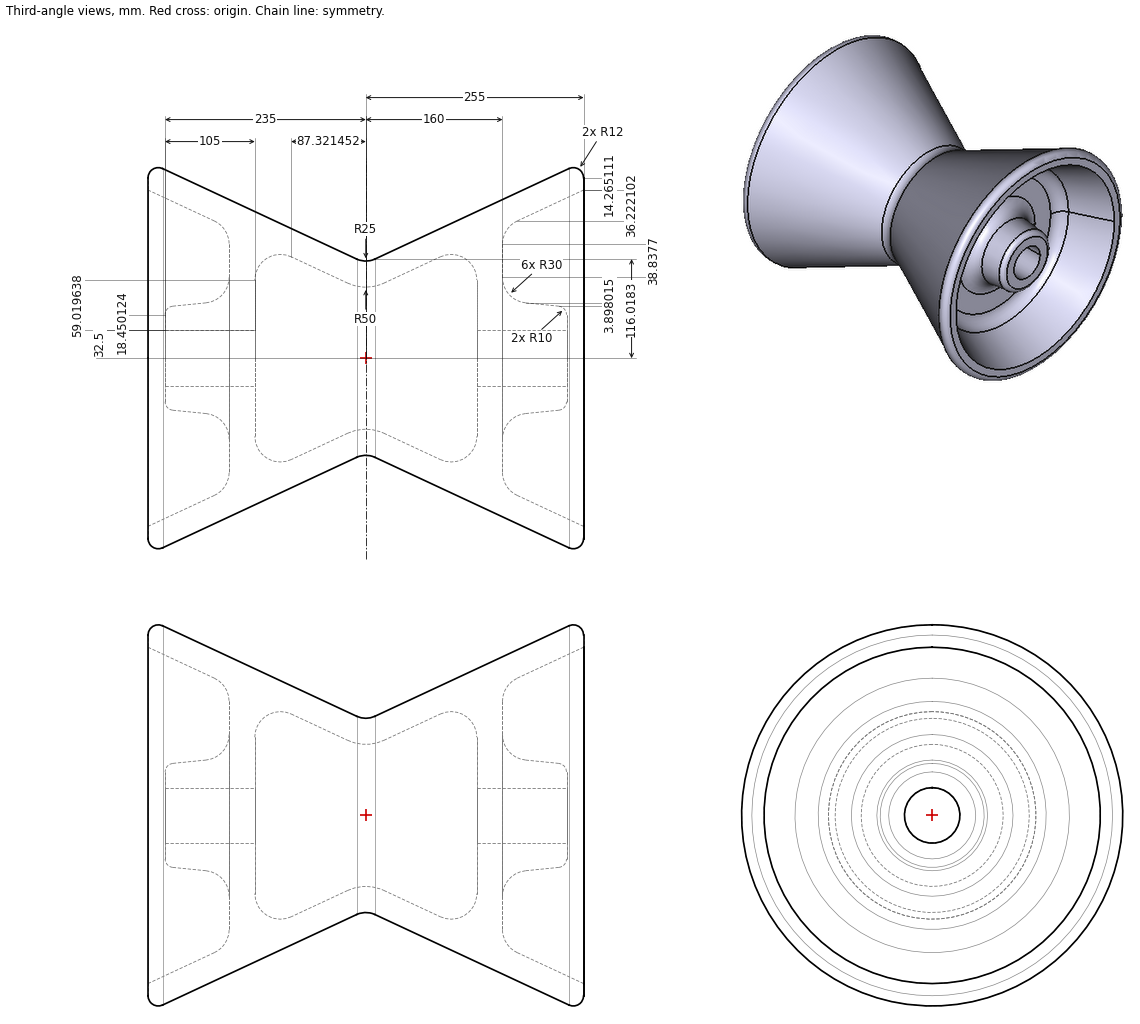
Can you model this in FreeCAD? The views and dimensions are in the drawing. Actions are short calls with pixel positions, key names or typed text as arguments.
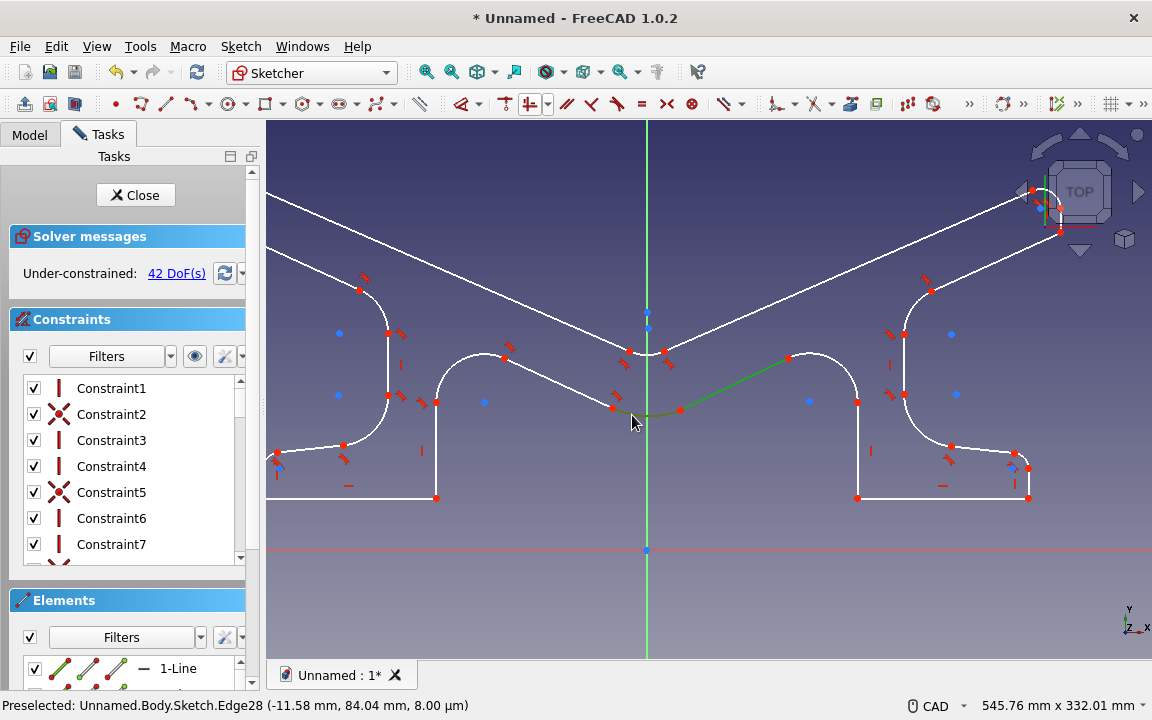
key(t)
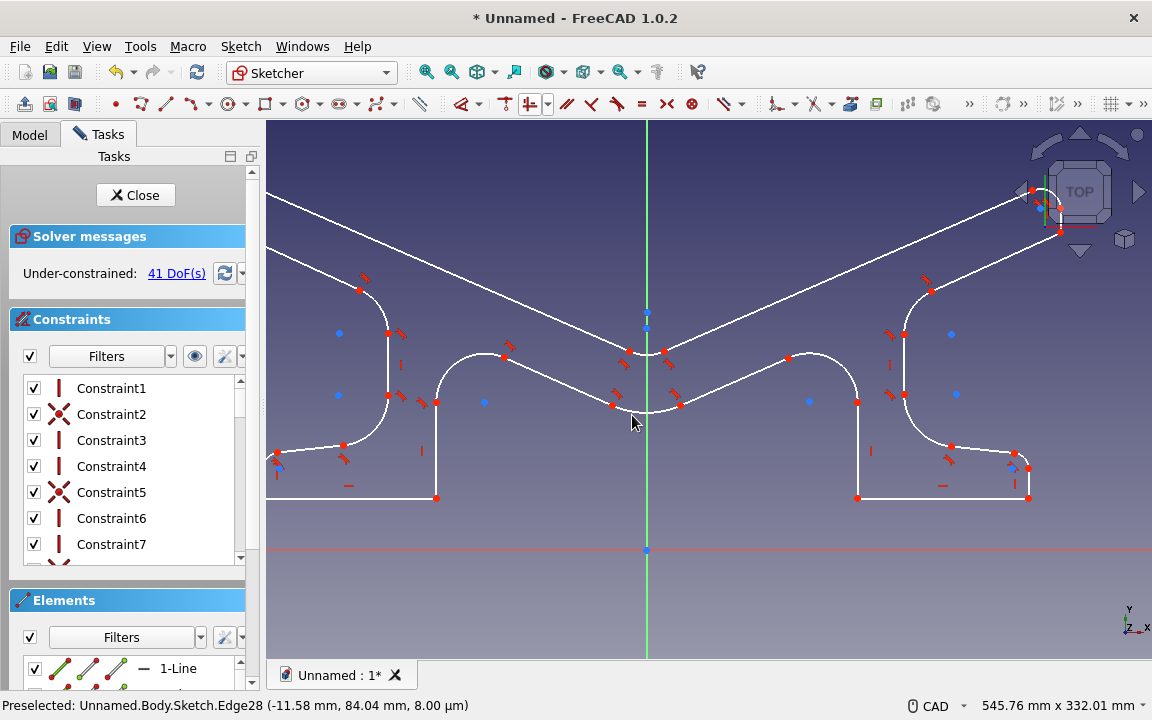
click(713, 391)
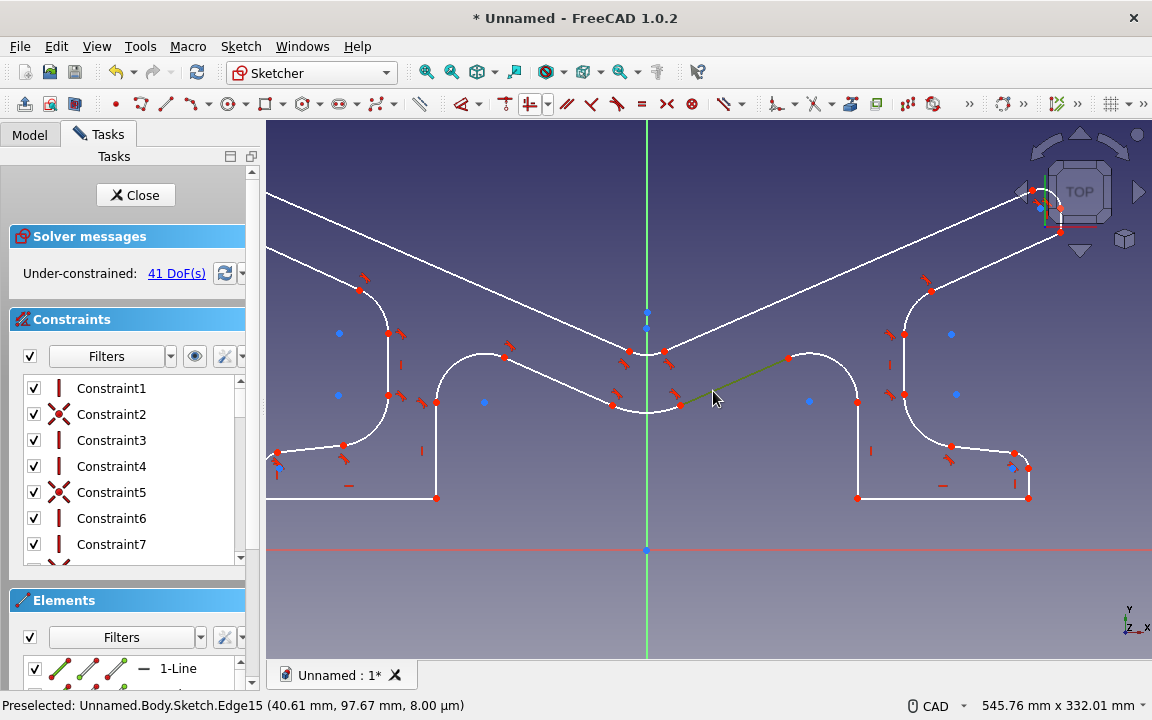
click(849, 374)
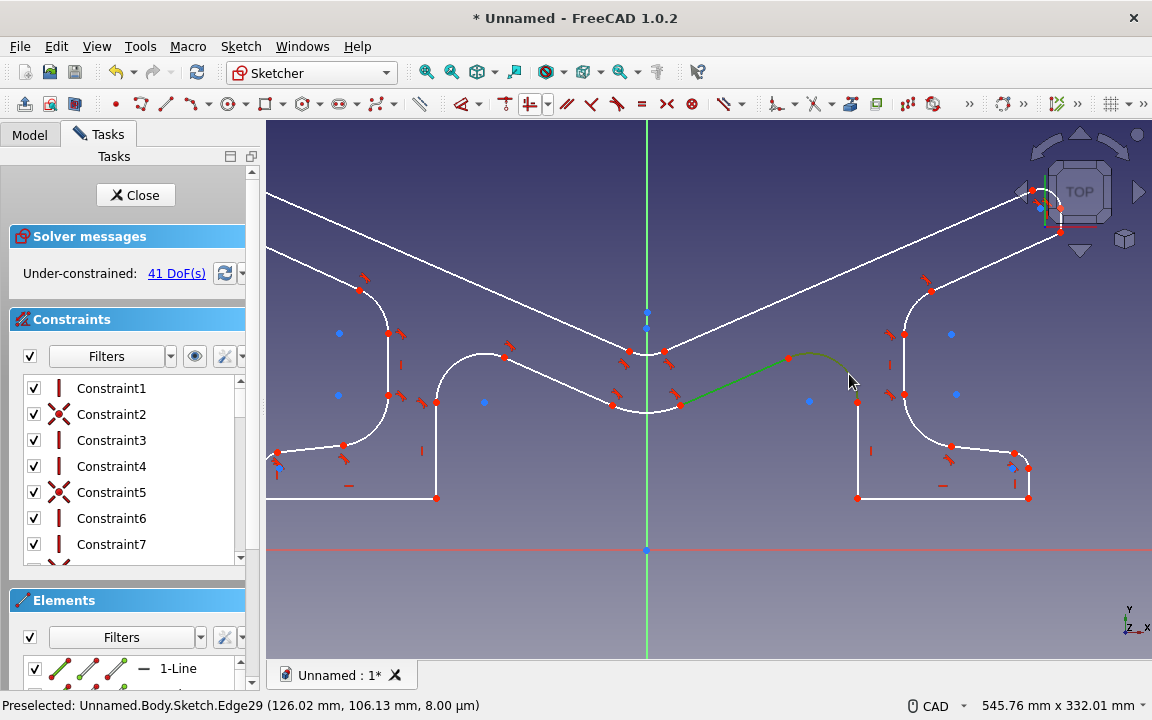
click(617, 104)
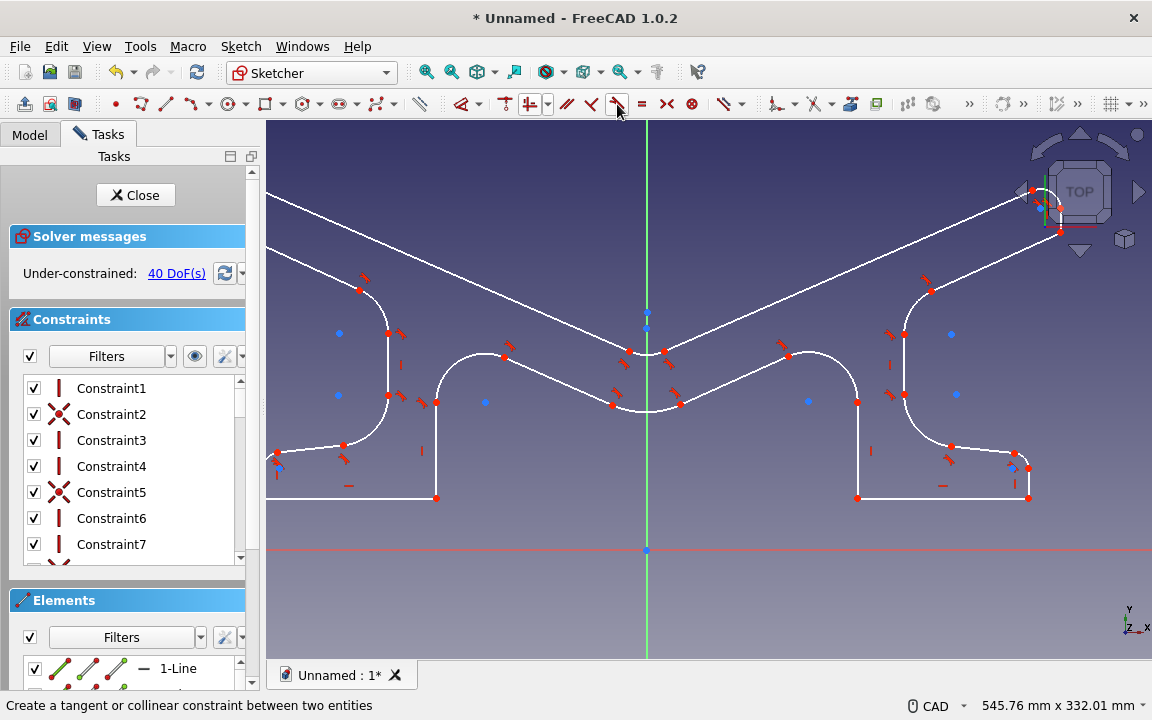
click(858, 431)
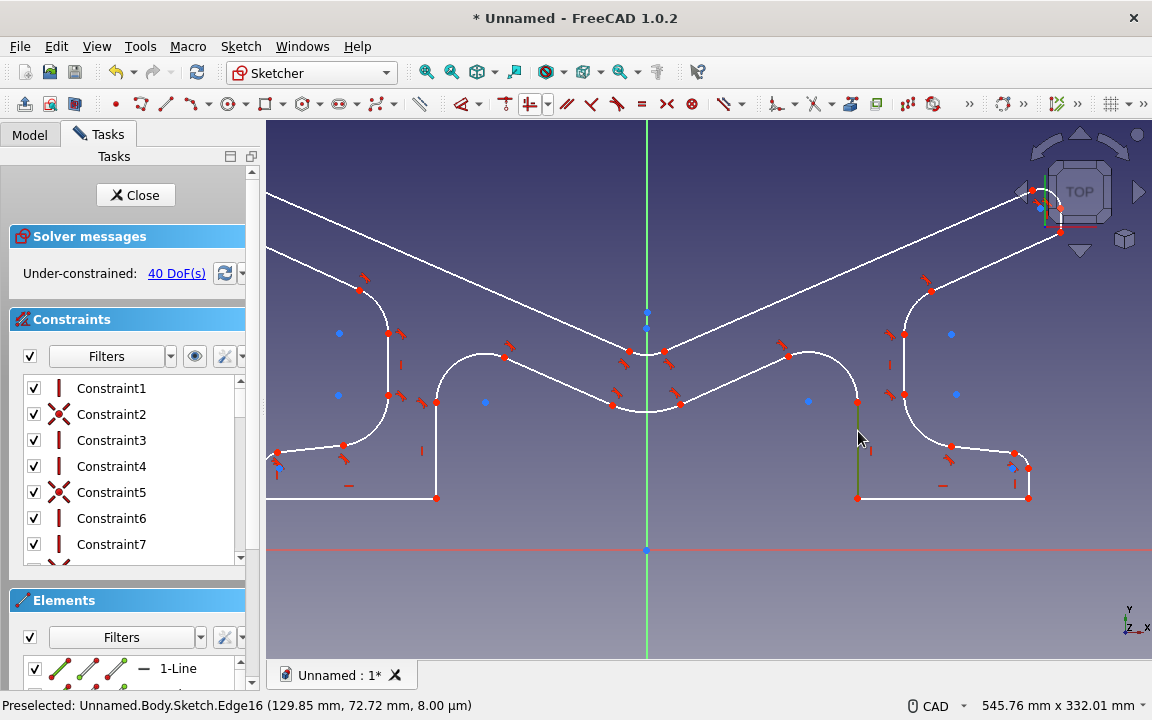
click(849, 374)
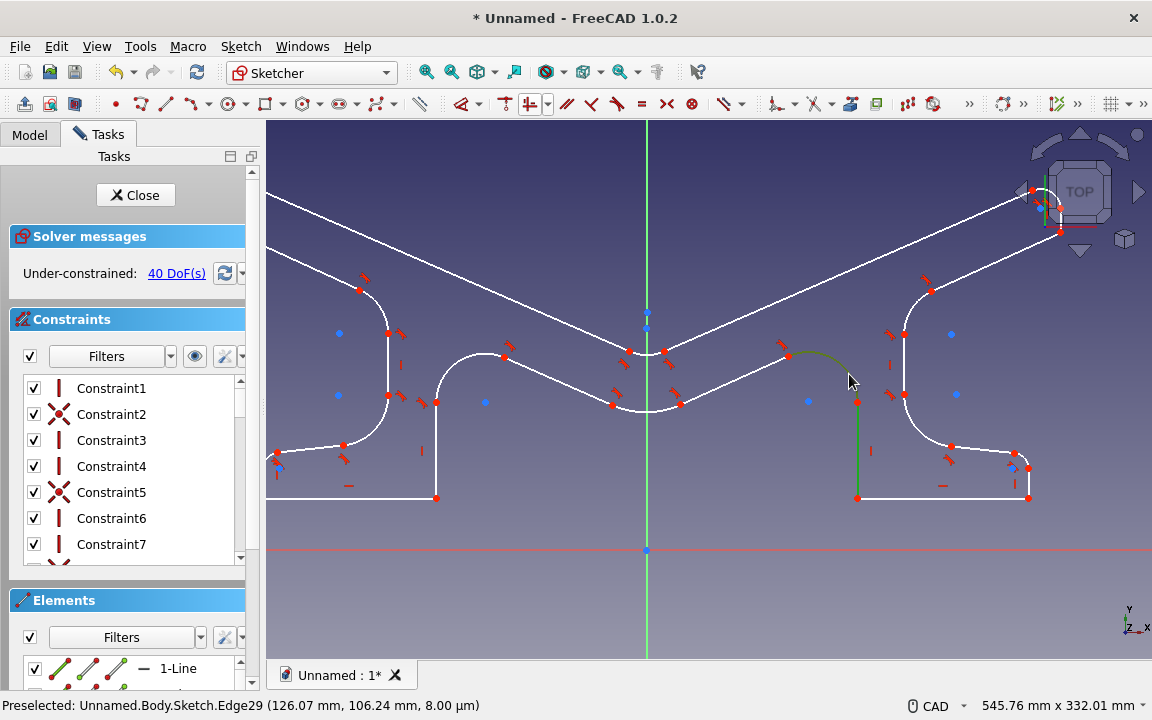
click(617, 104)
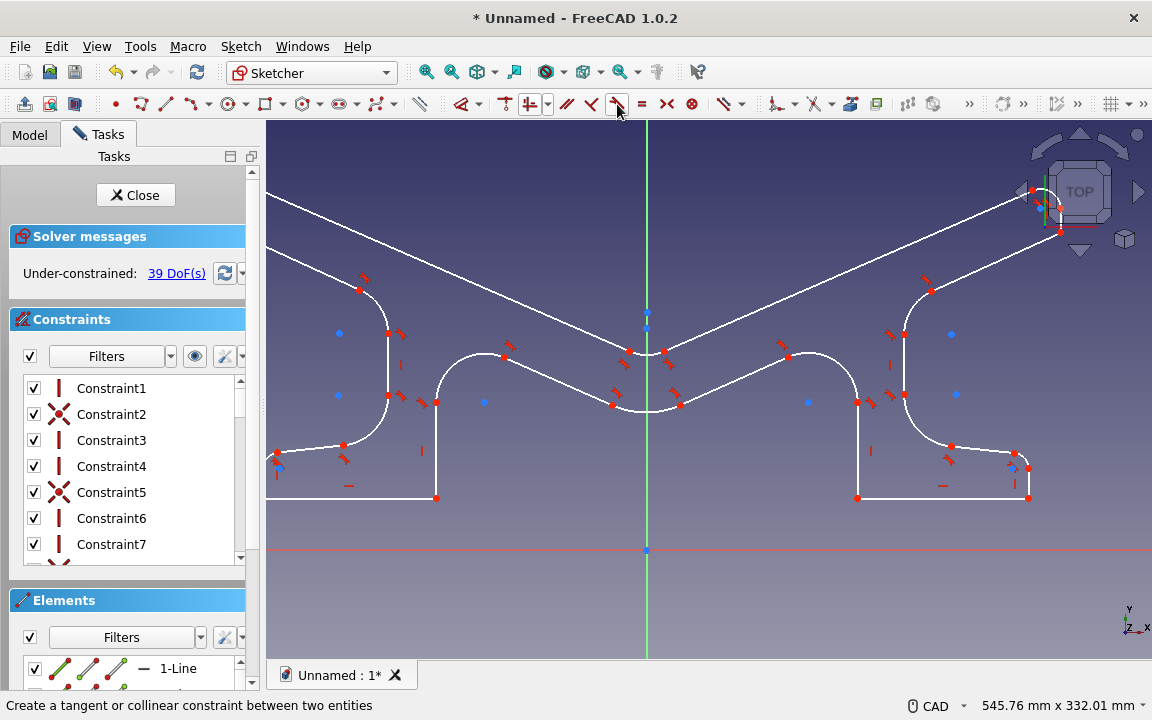
scroll(633, 413, down, 3)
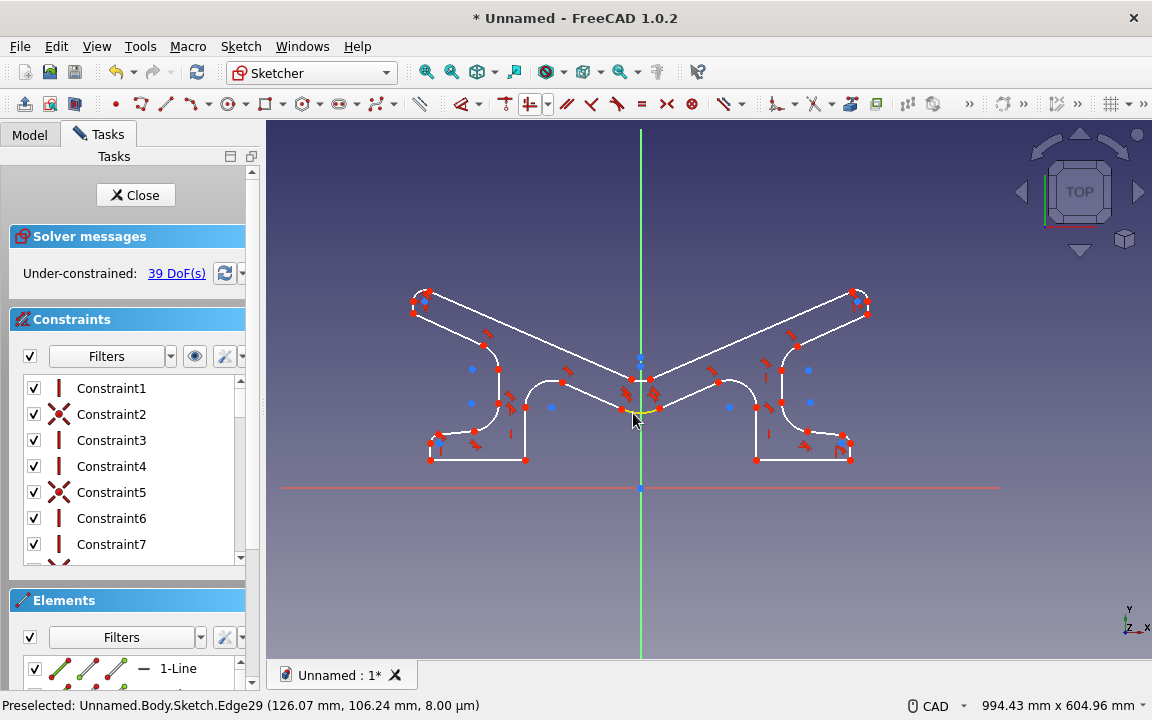
scroll(850, 455, up, 6)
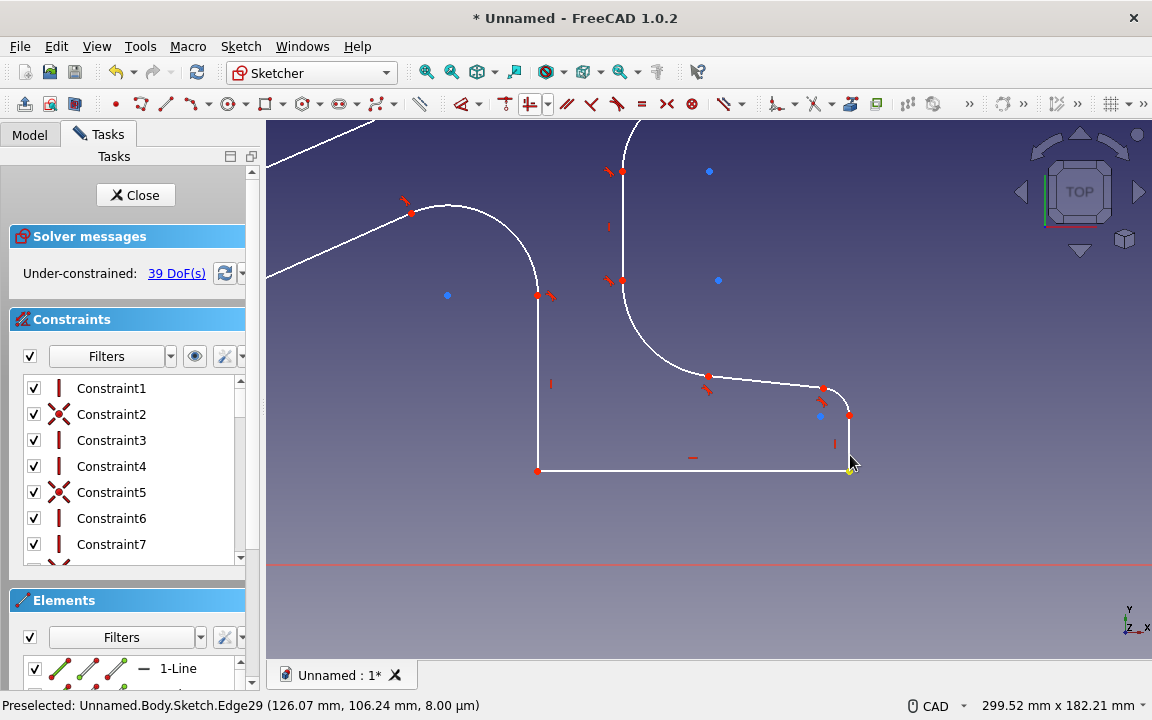
click(849, 455)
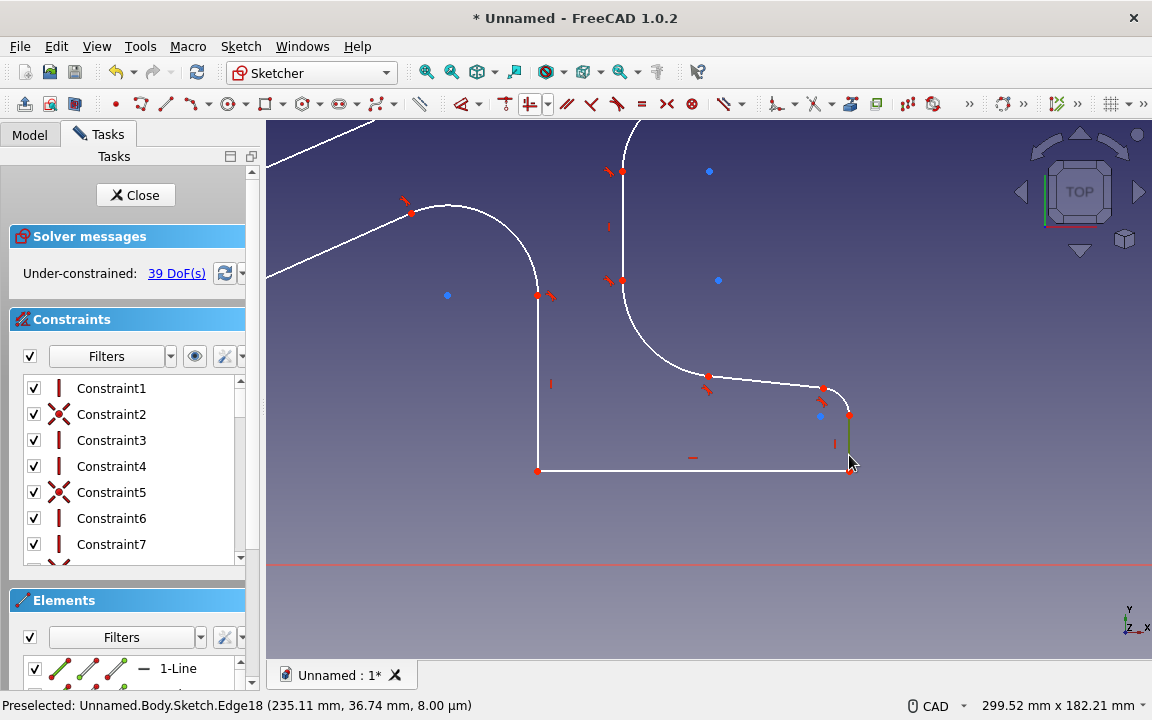
click(846, 404)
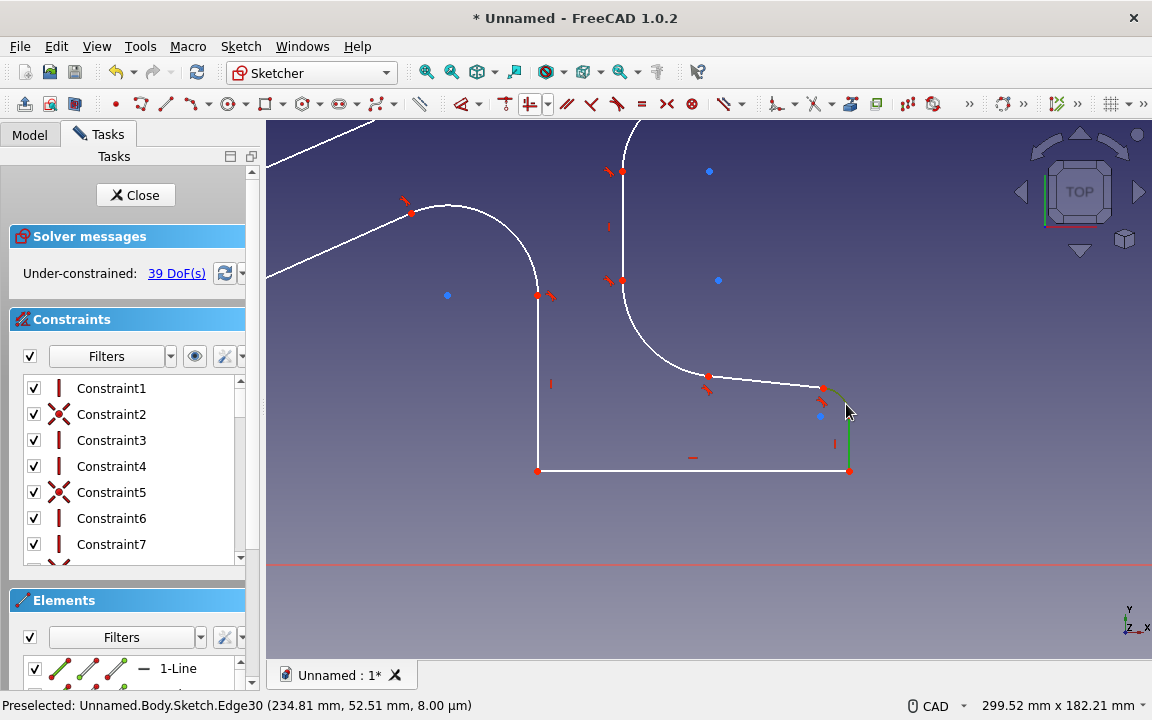
click(617, 104)